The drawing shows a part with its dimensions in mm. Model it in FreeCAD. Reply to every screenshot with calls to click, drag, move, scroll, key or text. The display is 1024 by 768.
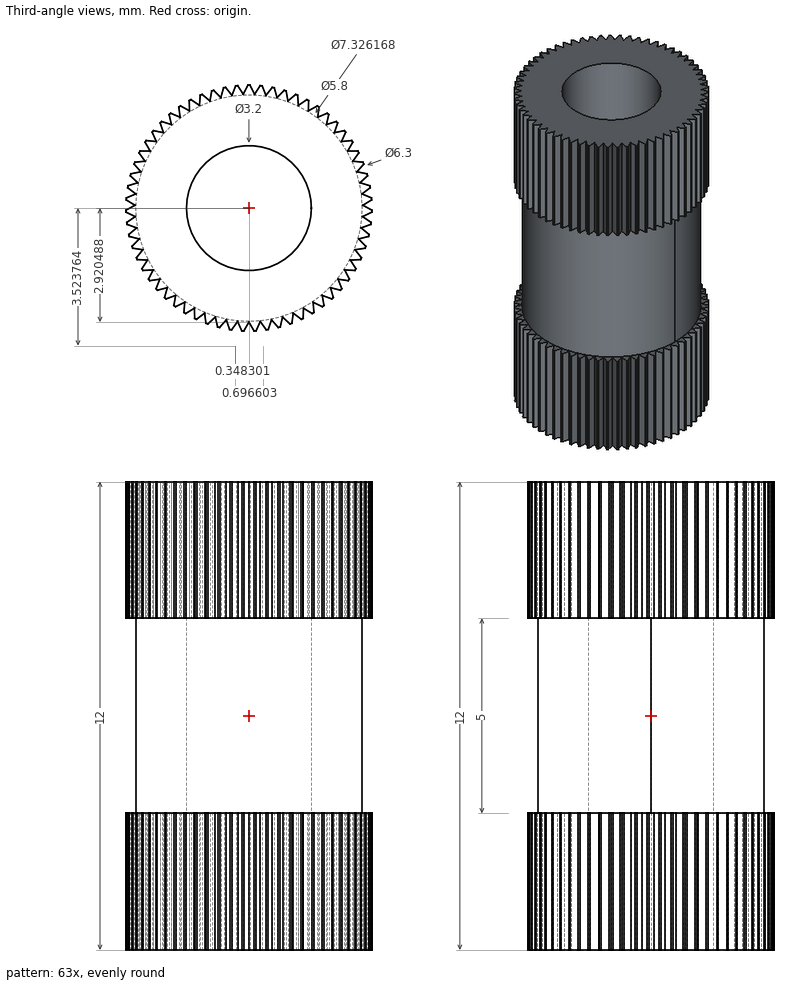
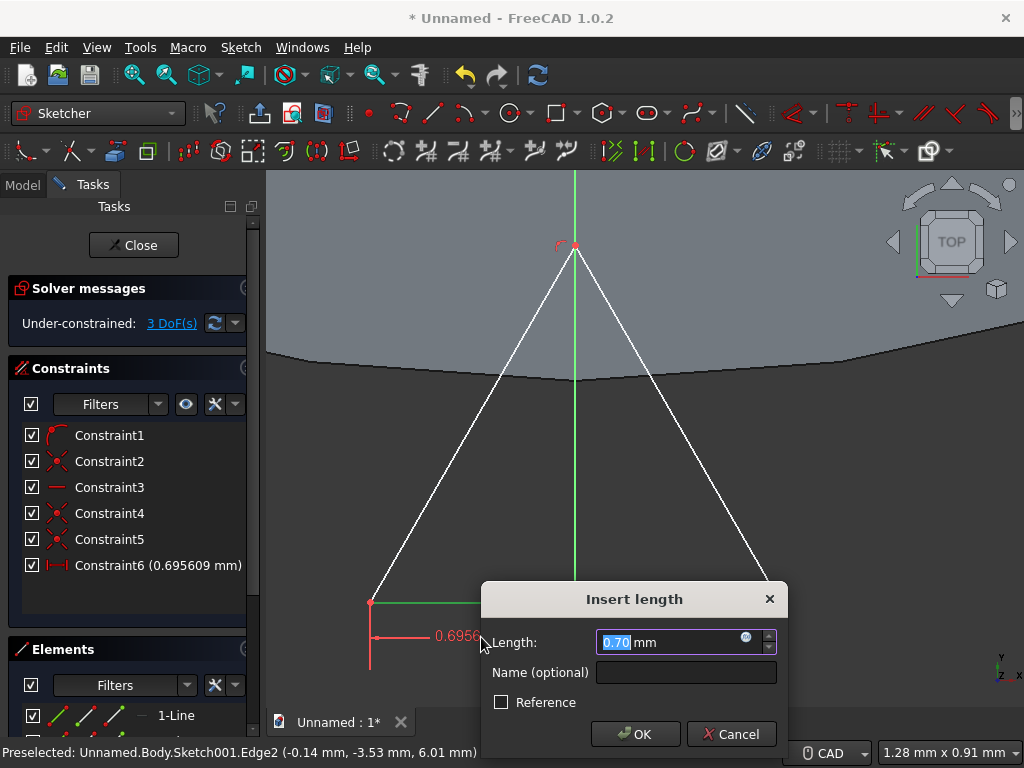
text(0.696603)
key(Return)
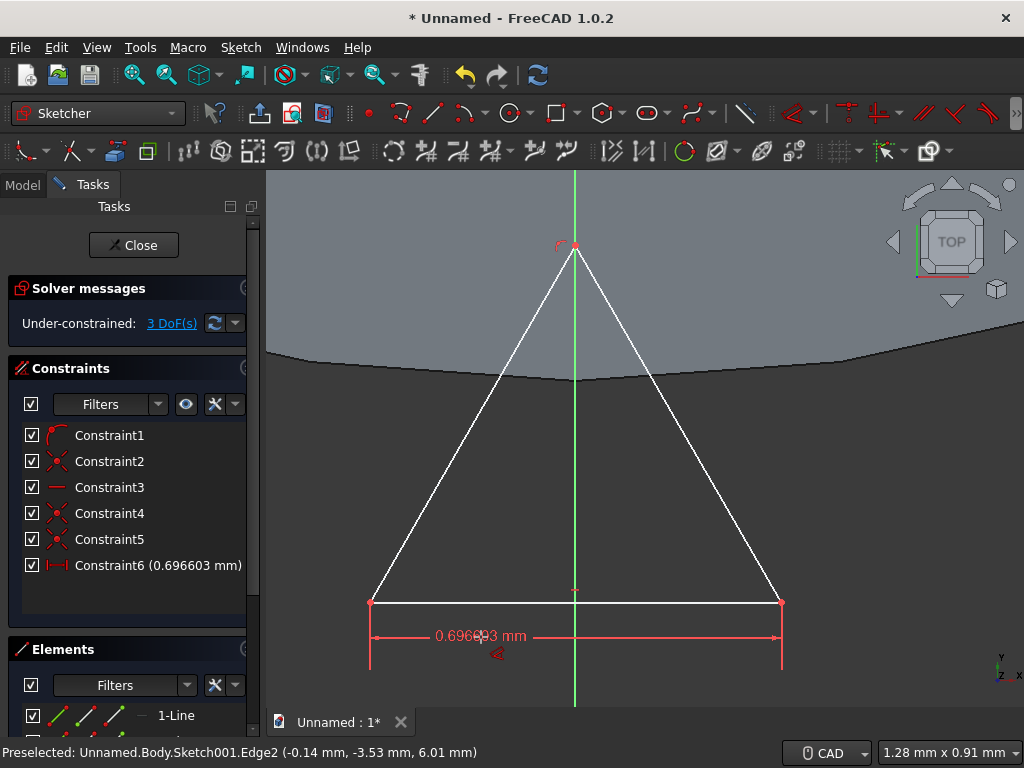
click(575, 246)
click(609, 222)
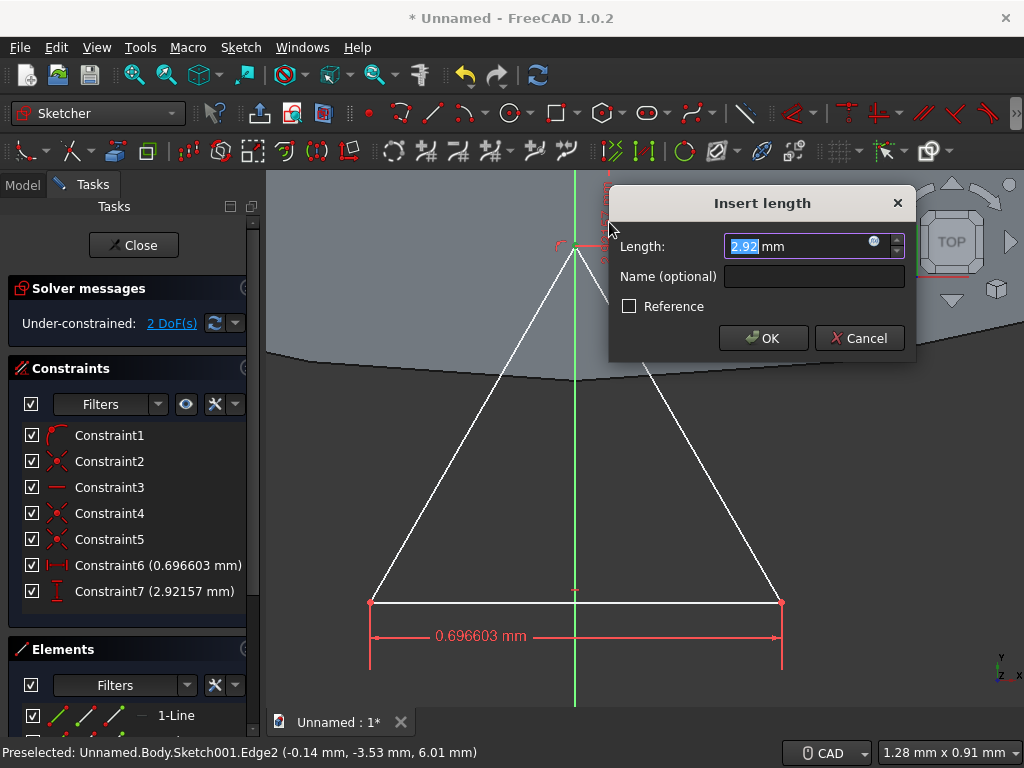
text(2.920488)
key(Return)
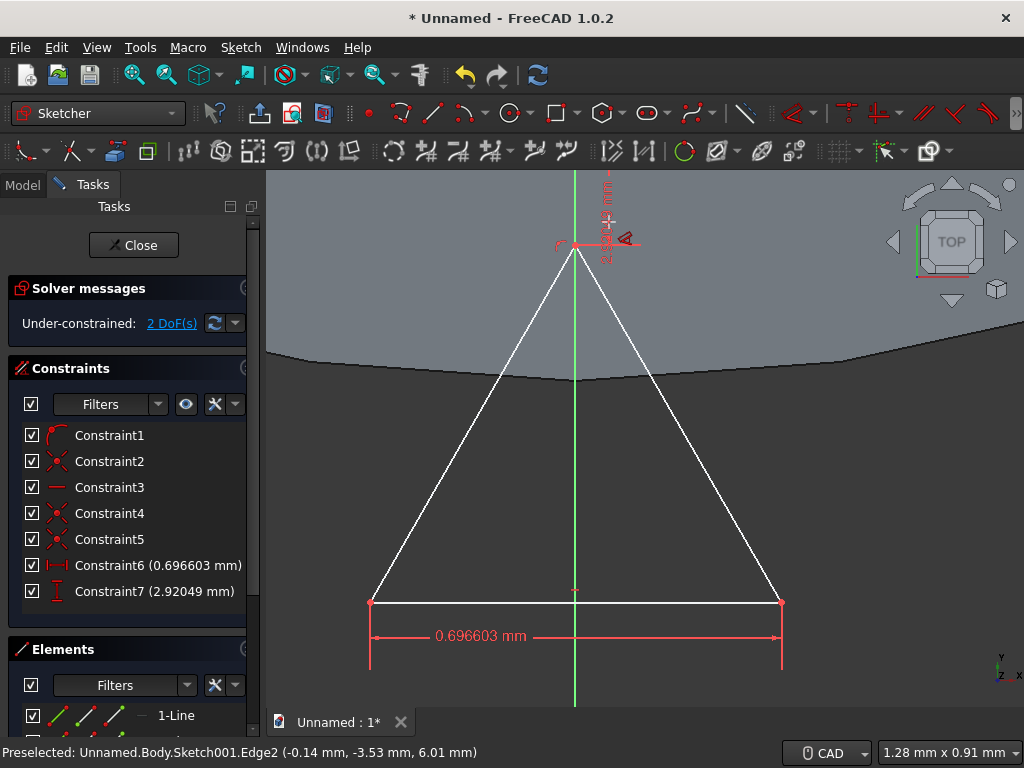
click(370, 603)
click(401, 637)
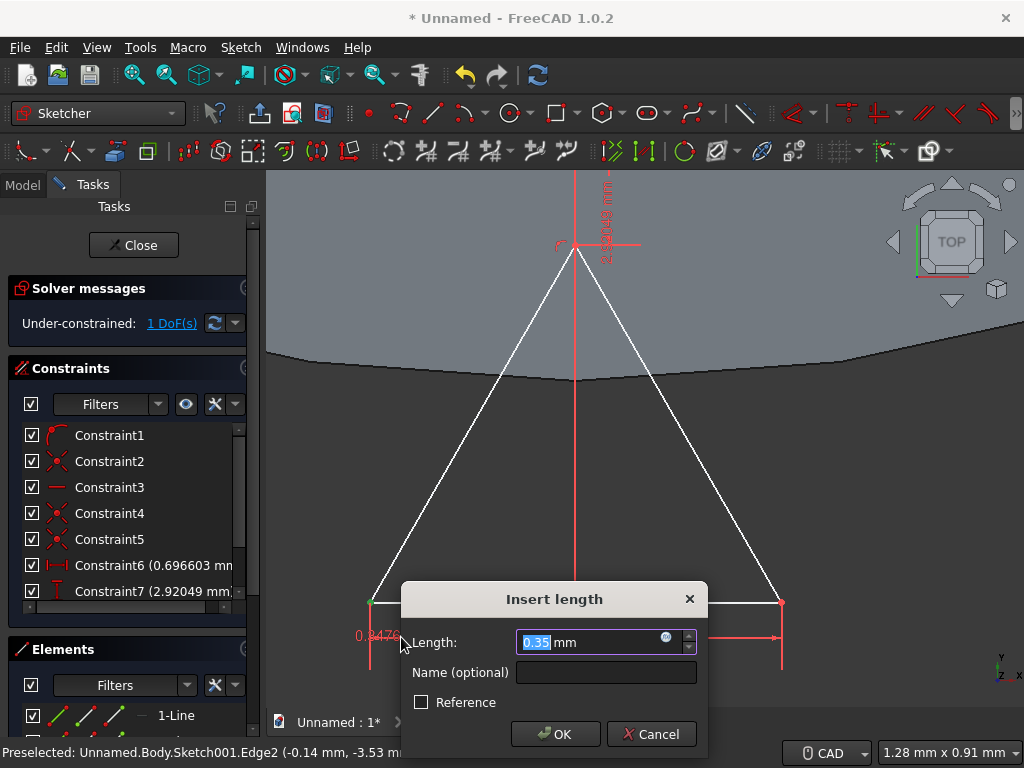
text(0.348301)
key(Return)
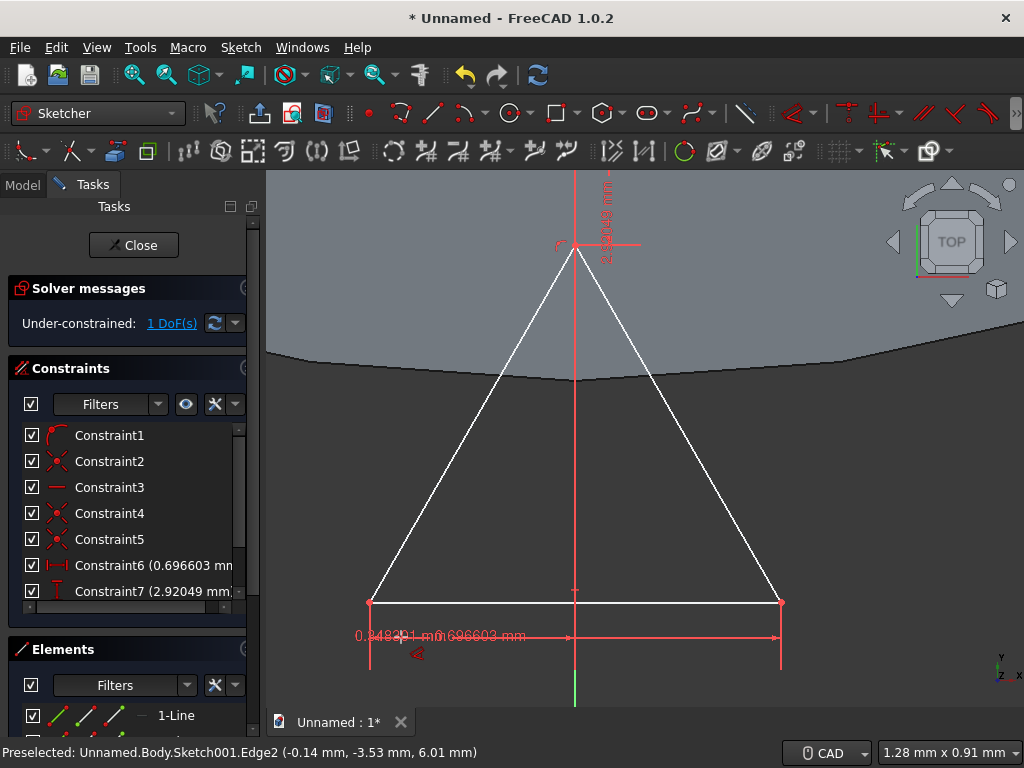
click(370, 603)
click(336, 400)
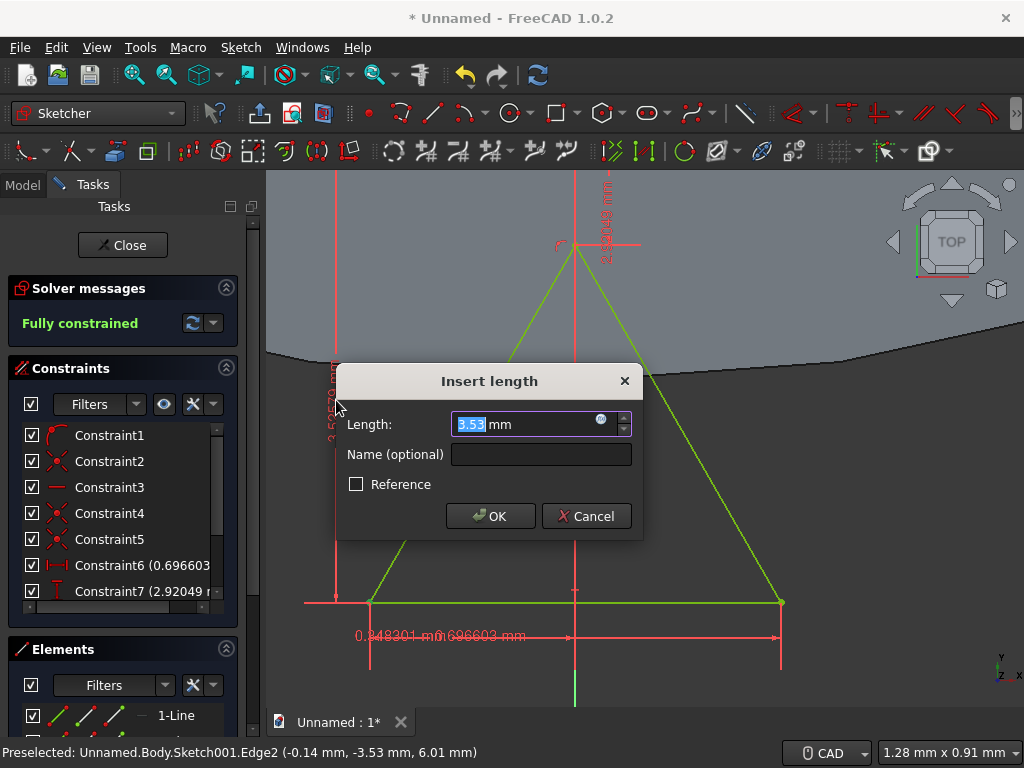
text(3.523764)
key(Return)
key(Escape)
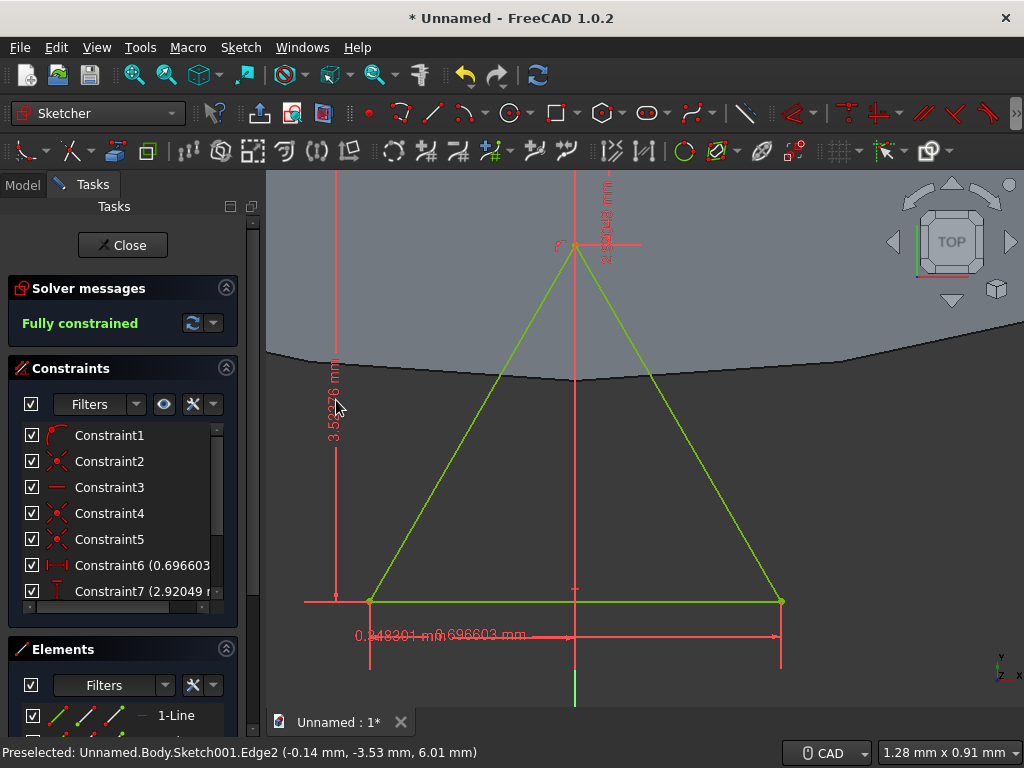
click(123, 245)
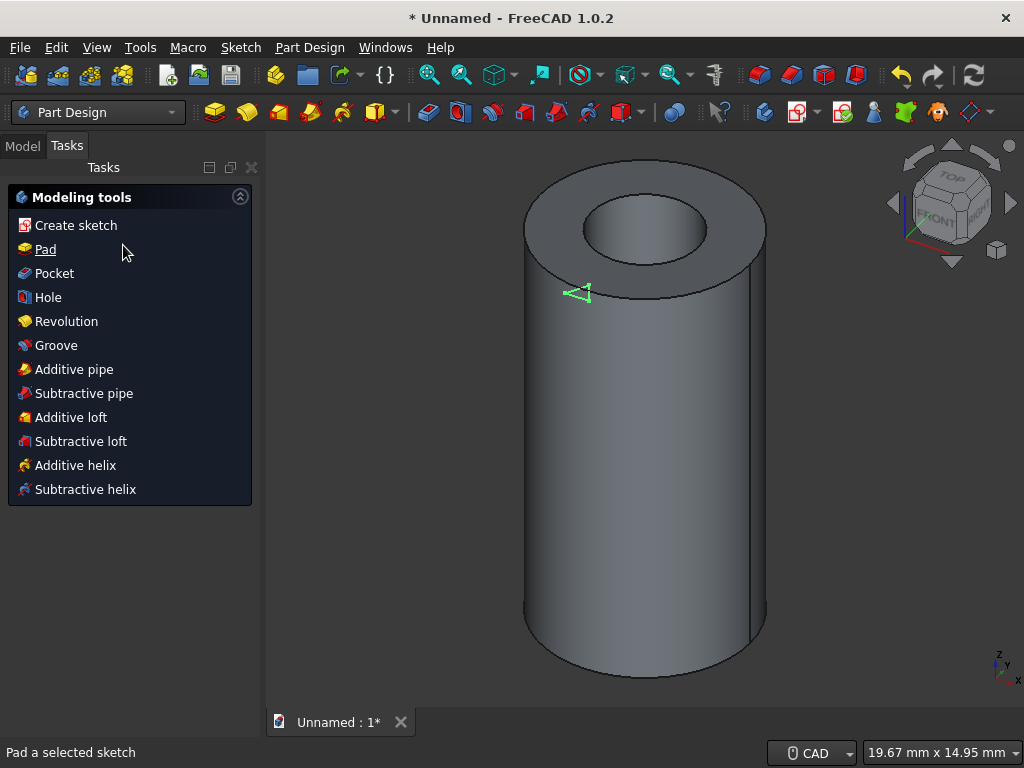
click(430, 112)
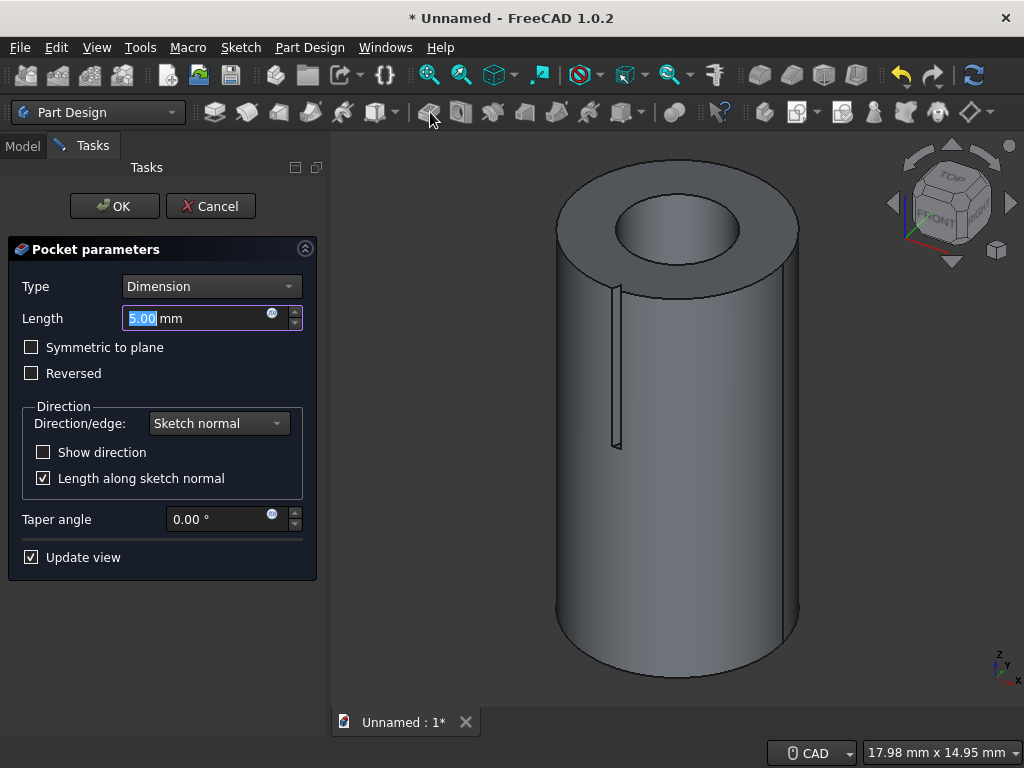
text(12)
key(Tab)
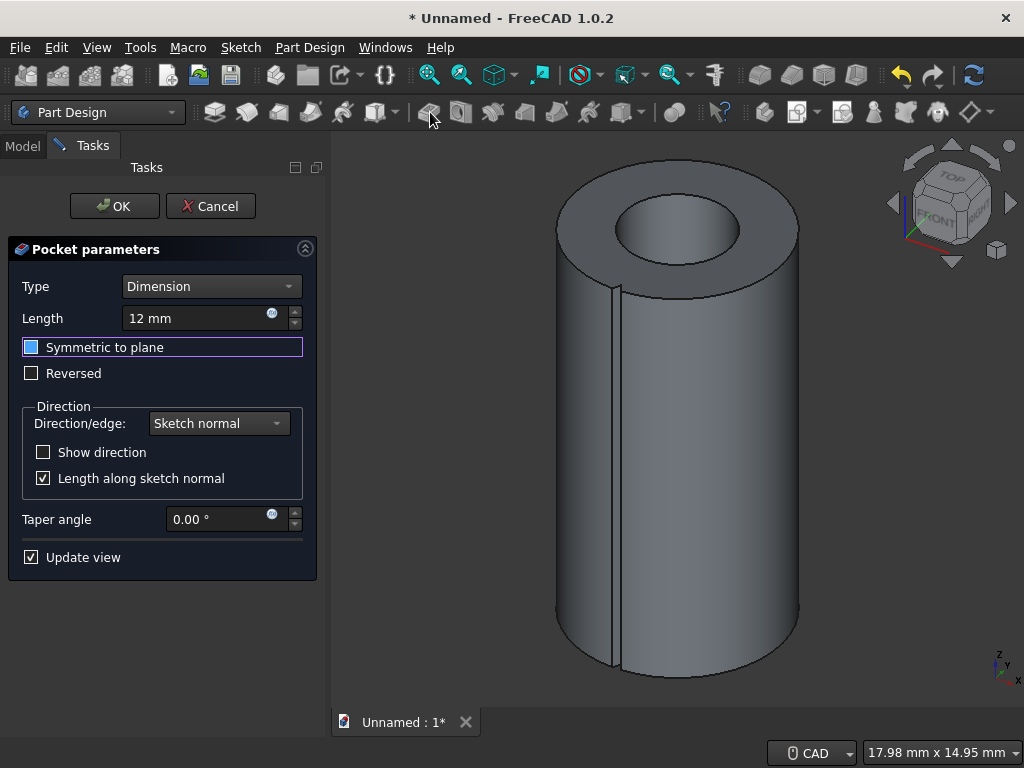
click(115, 206)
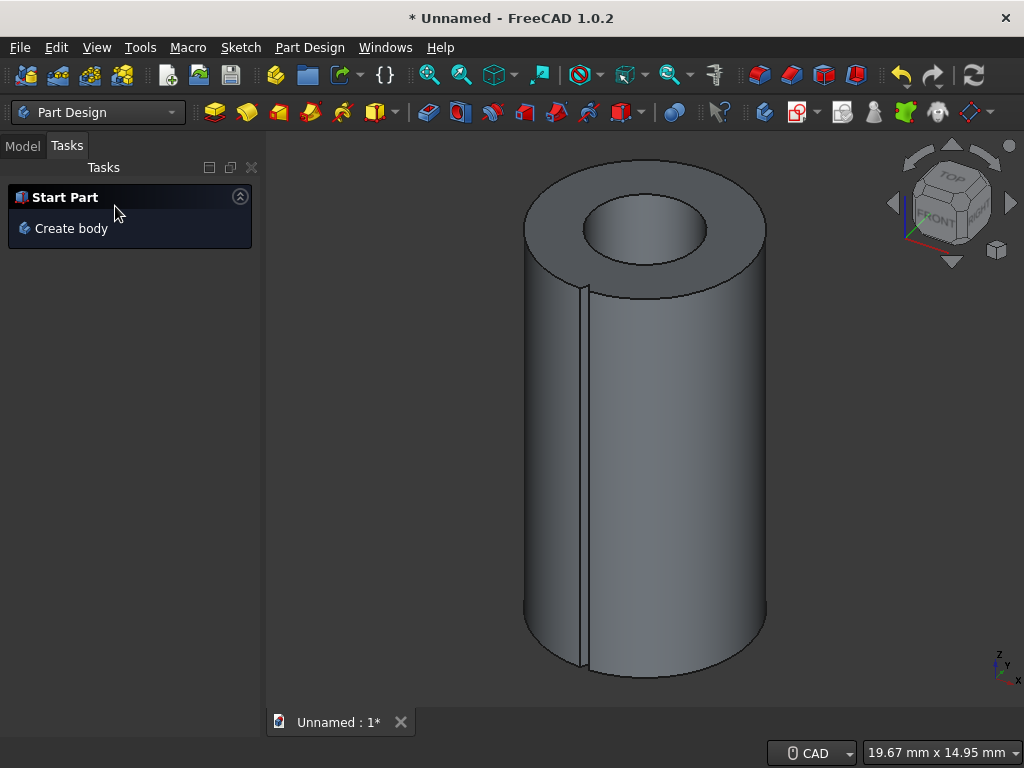
click(23, 145)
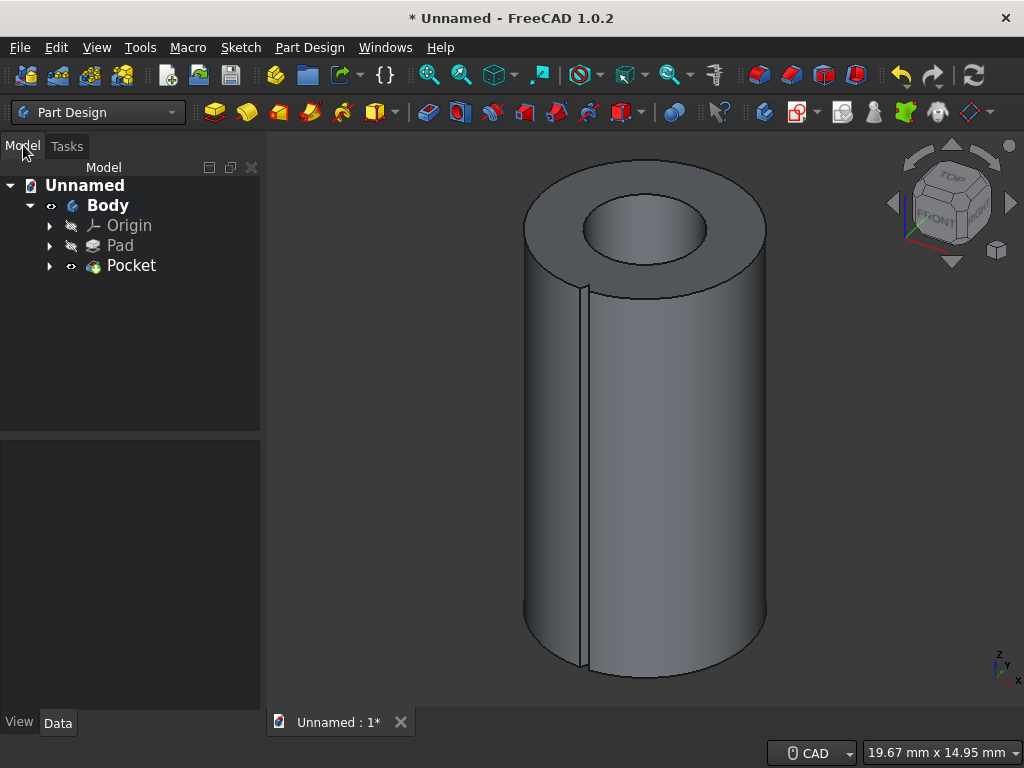
click(116, 266)